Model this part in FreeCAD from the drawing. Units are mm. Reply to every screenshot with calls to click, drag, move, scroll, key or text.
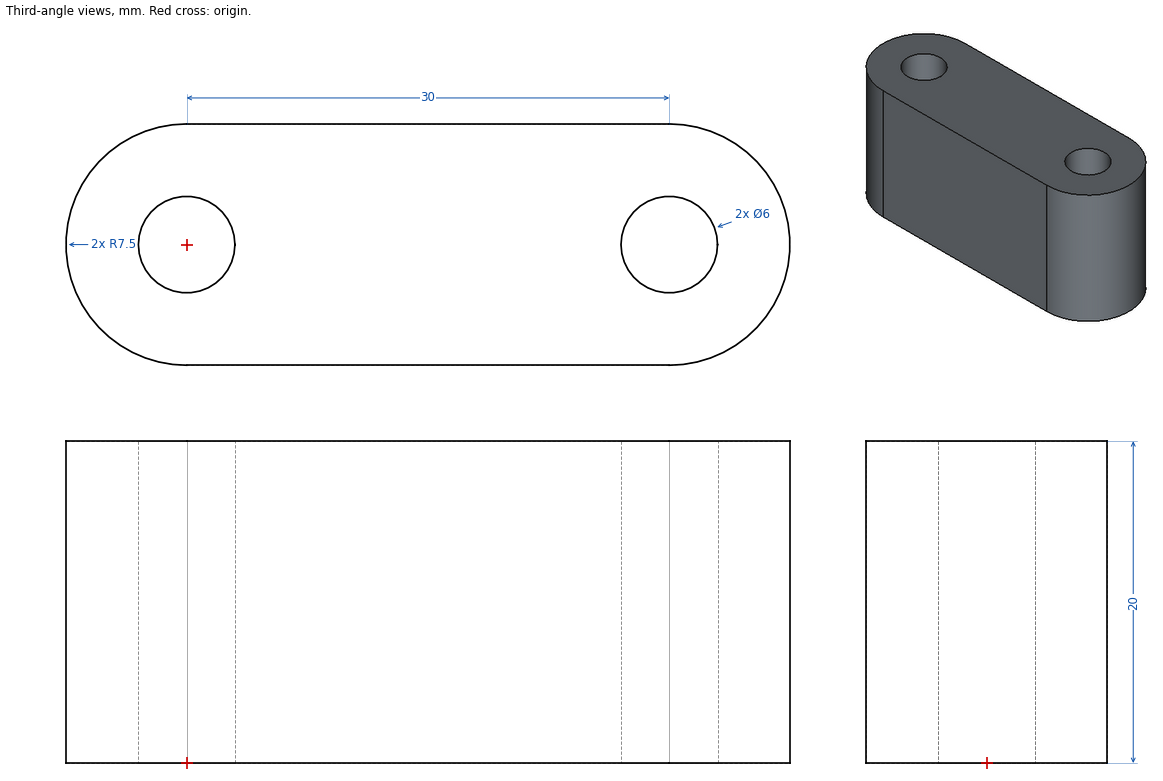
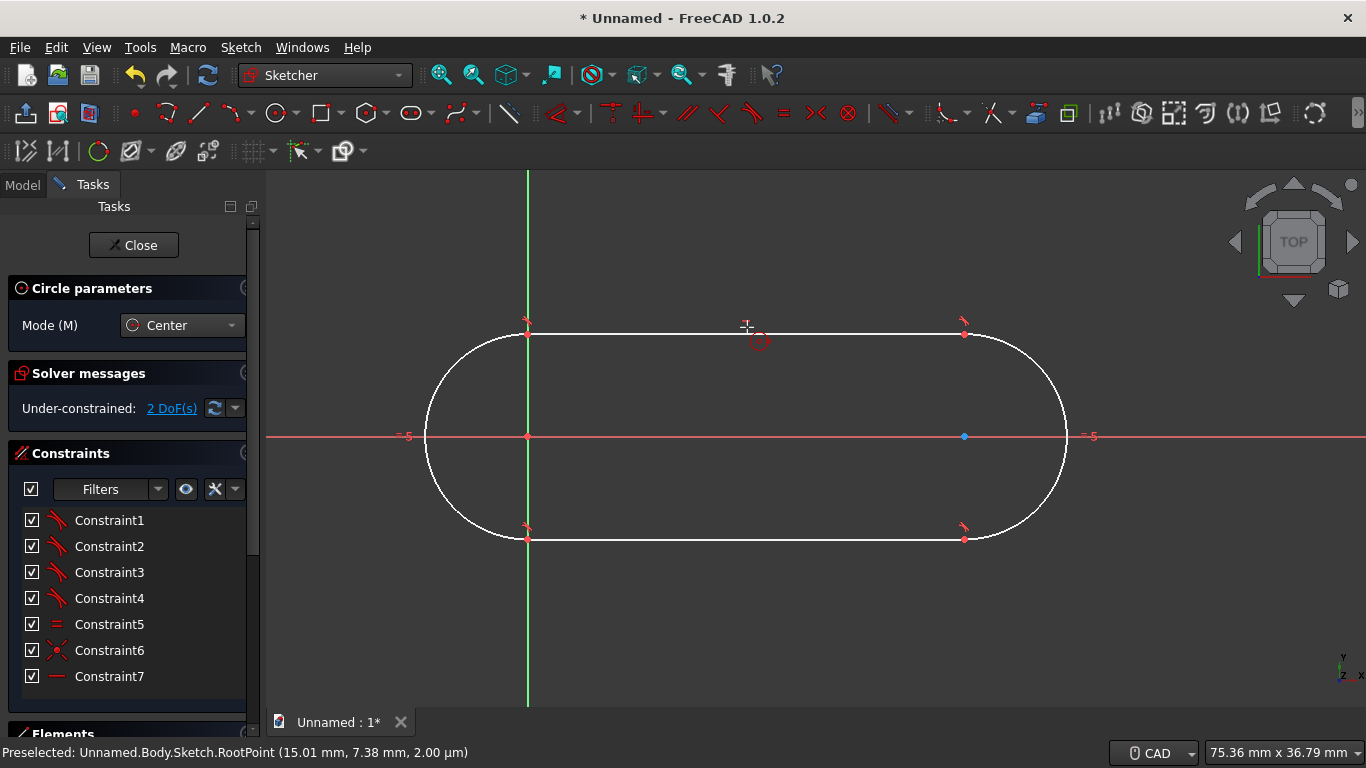
click(964, 437)
click(997, 406)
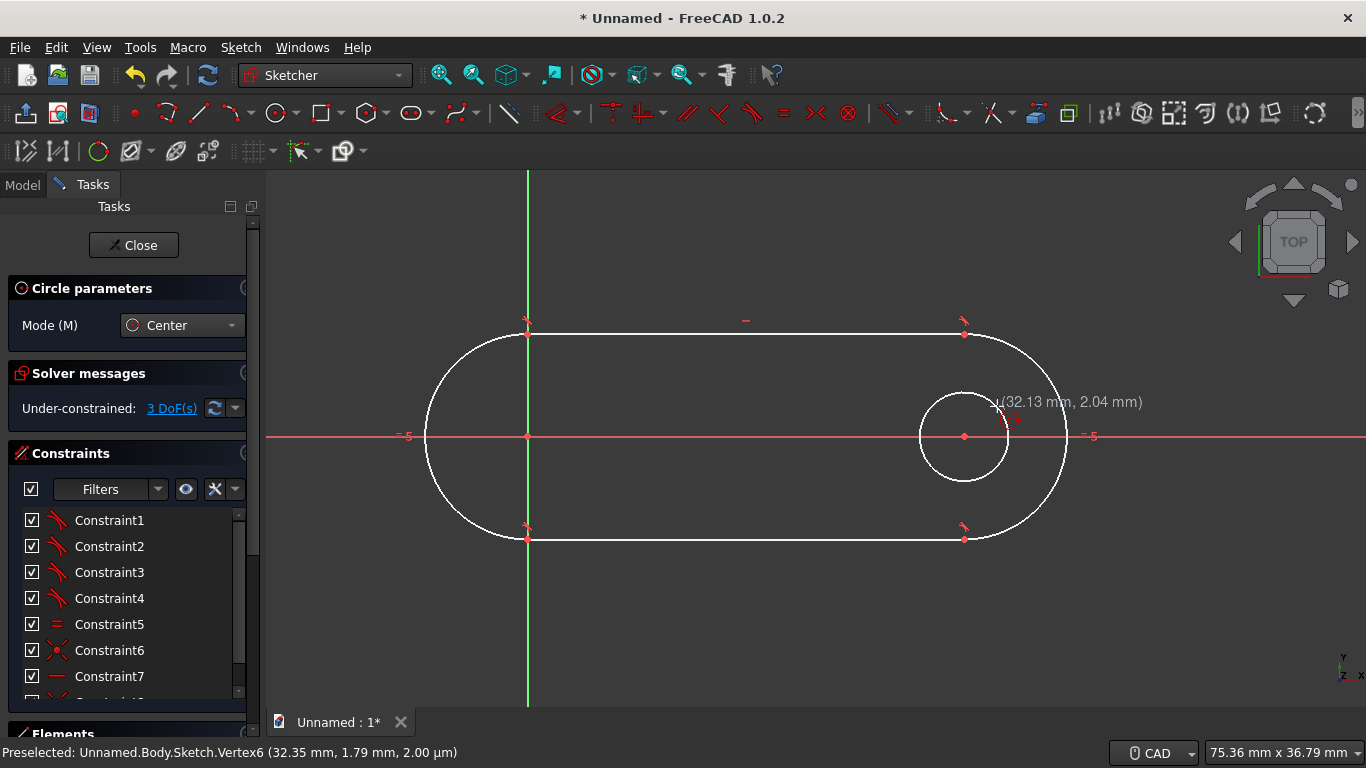
click(528, 437)
click(559, 406)
key(Escape)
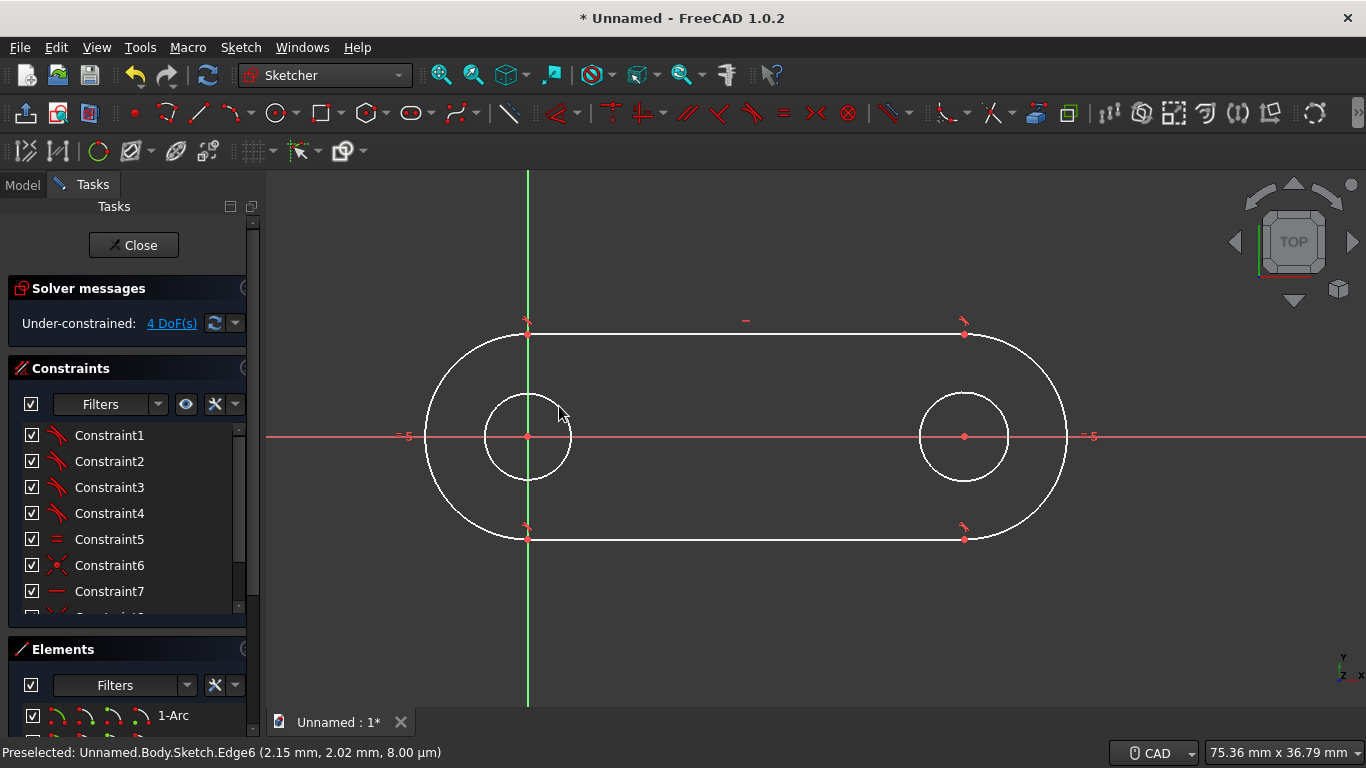
click(995, 405)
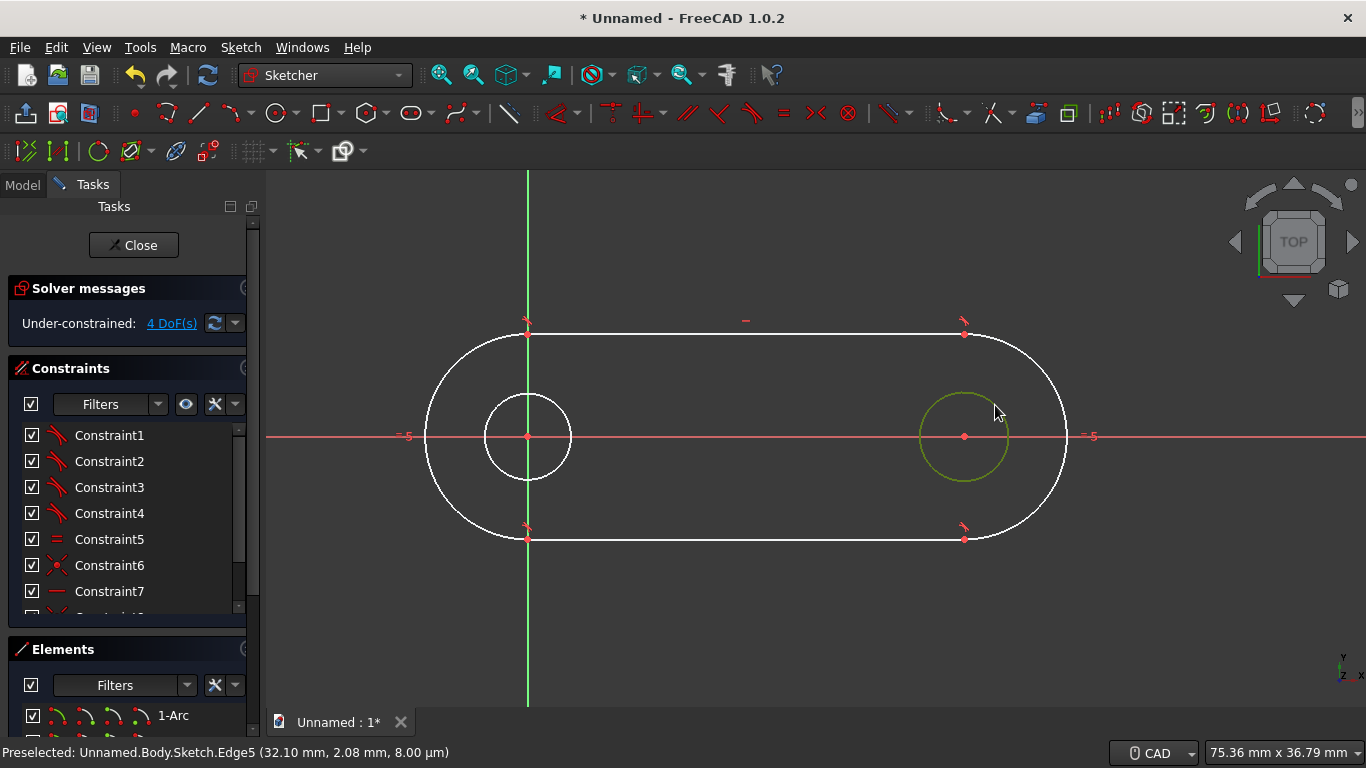
click(558, 406)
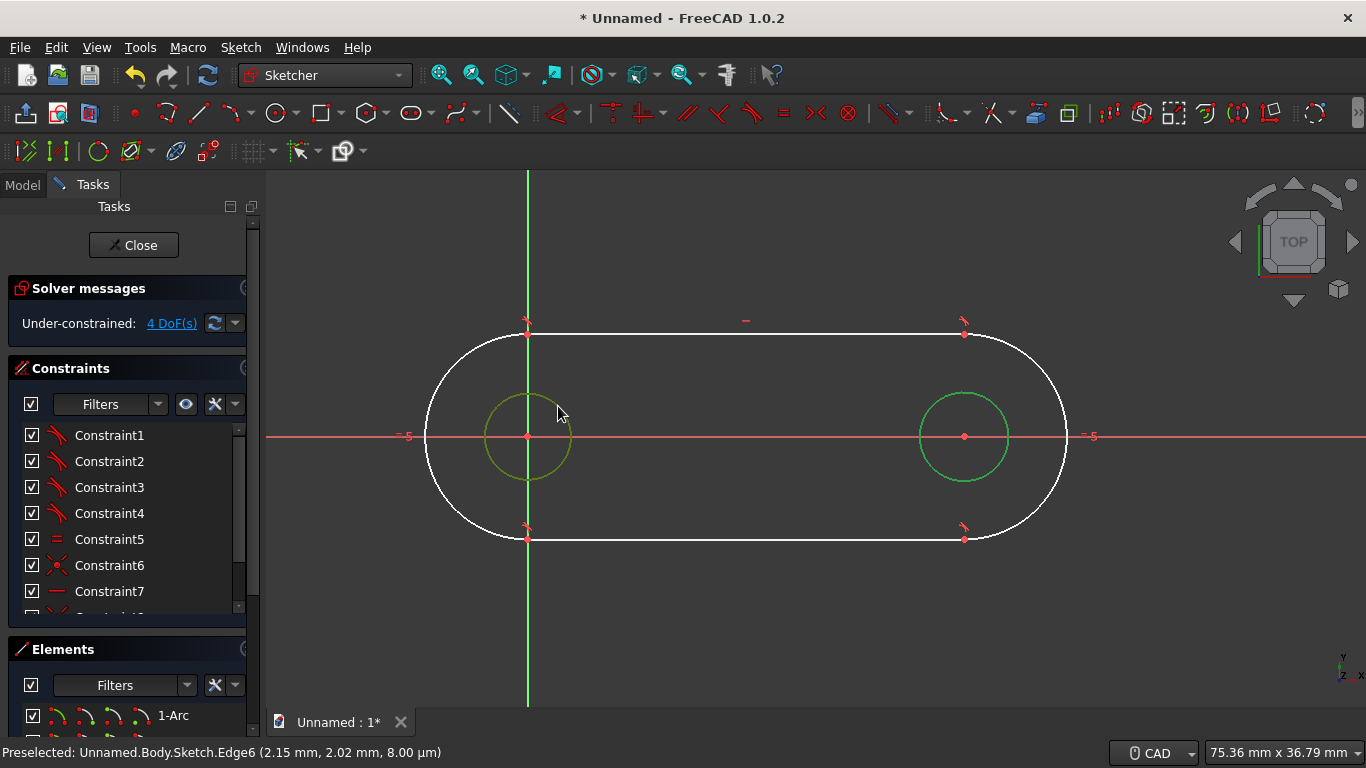
key(e)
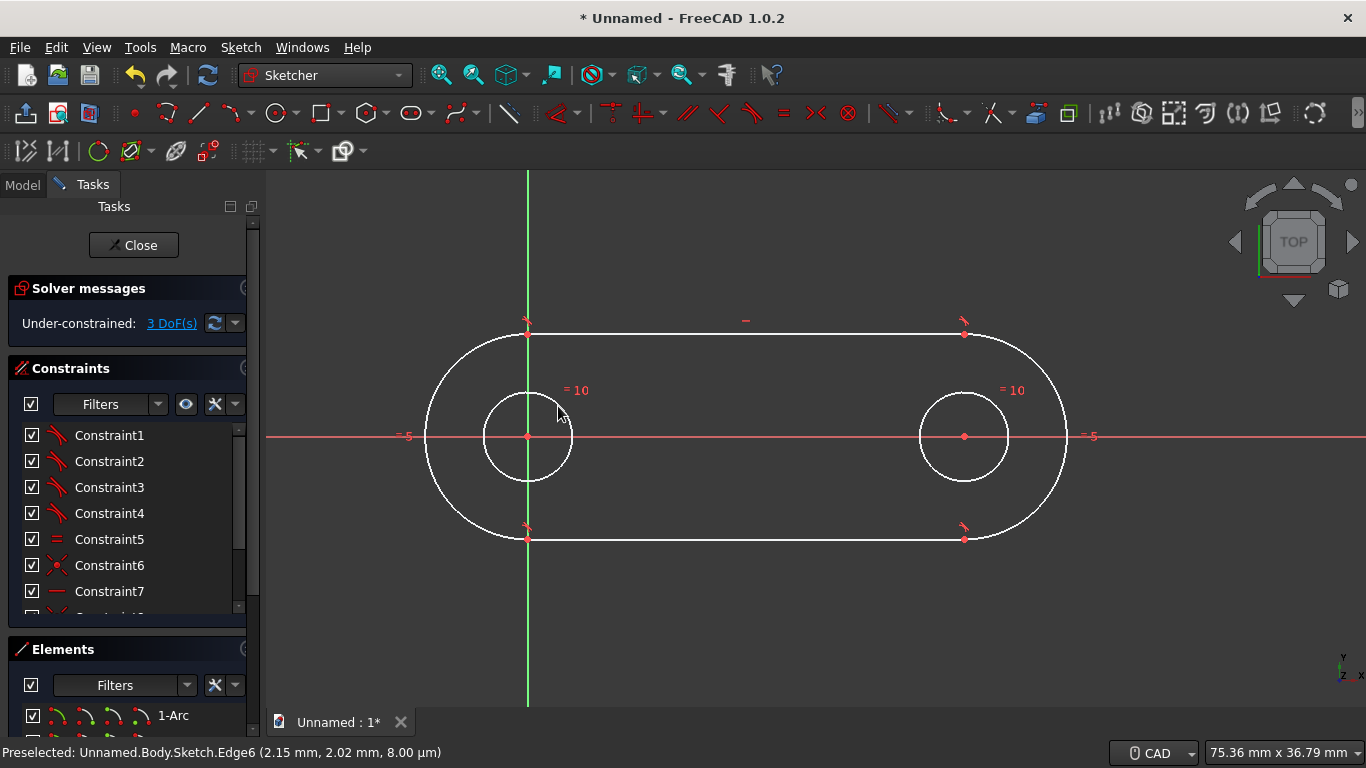
key(d)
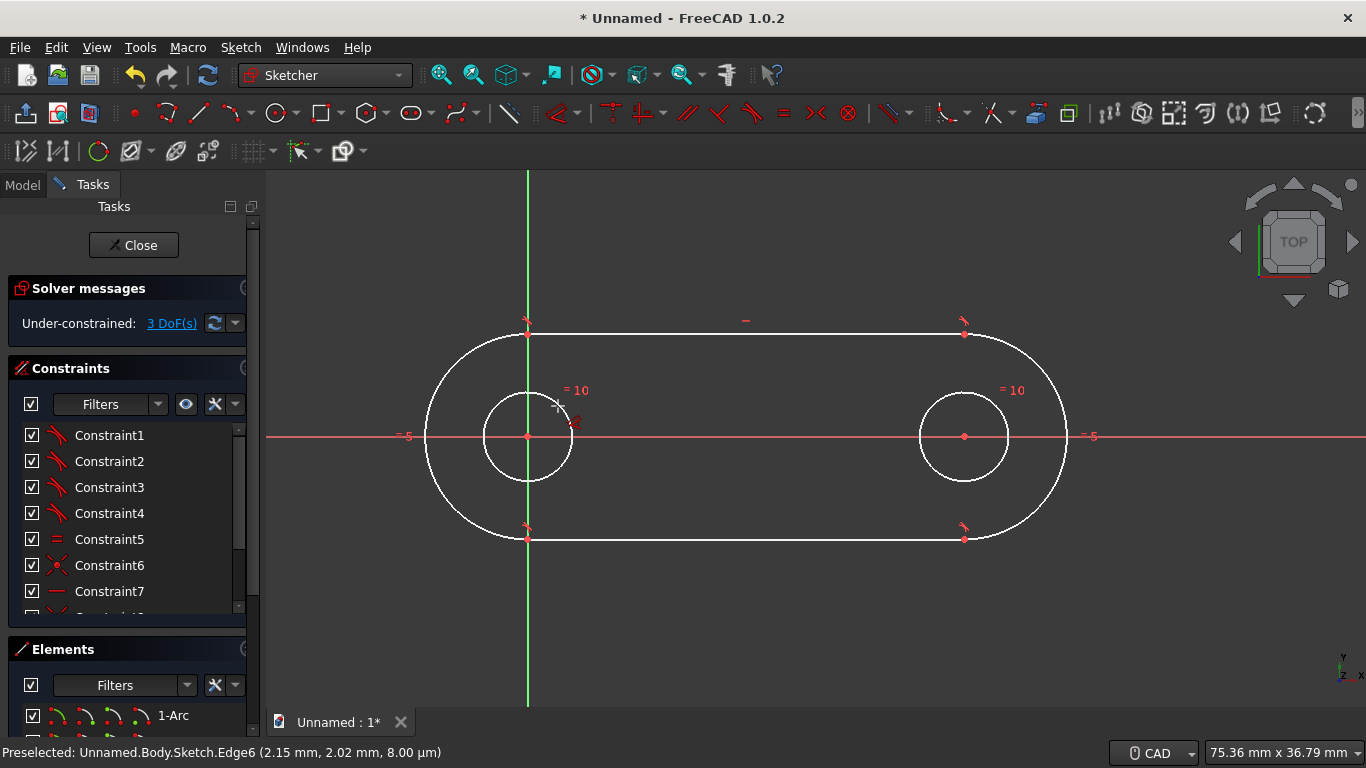
click(445, 376)
click(419, 357)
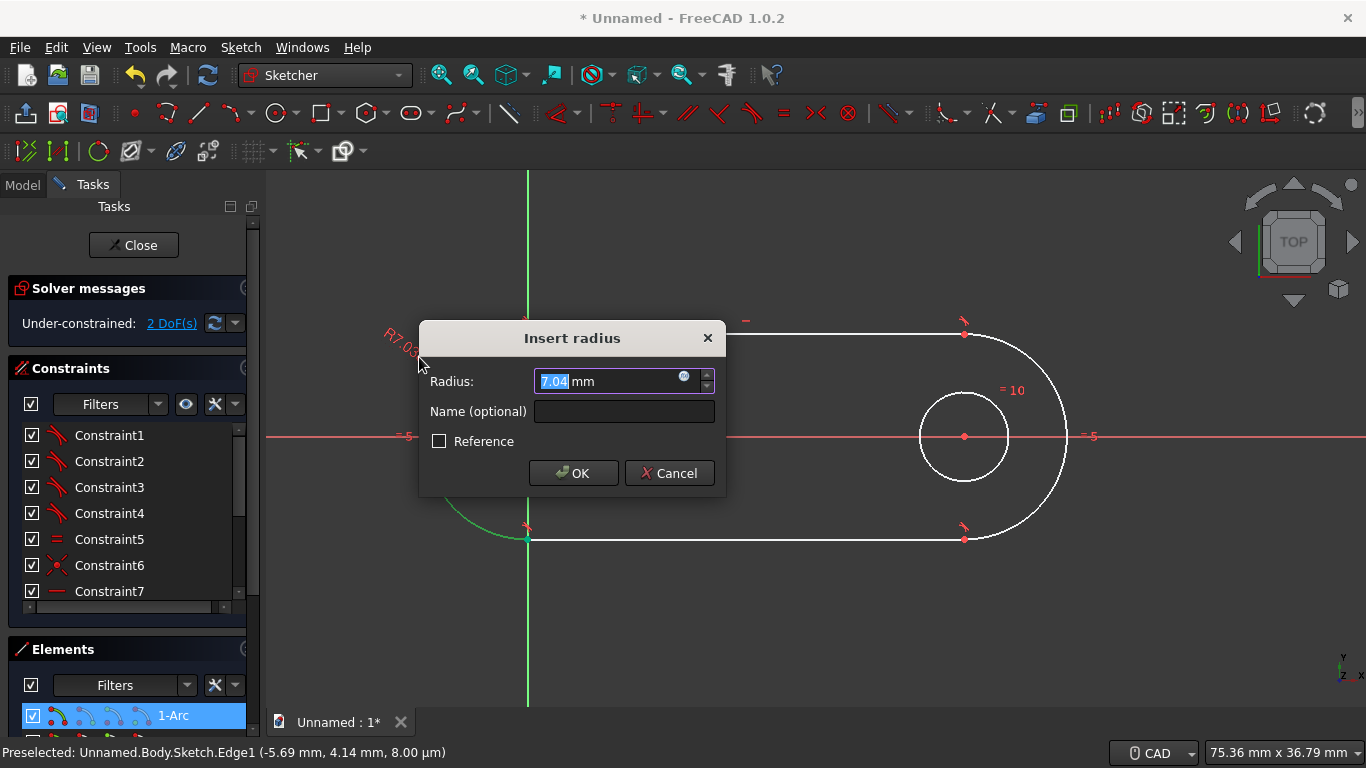
text(7.5)
key(Return)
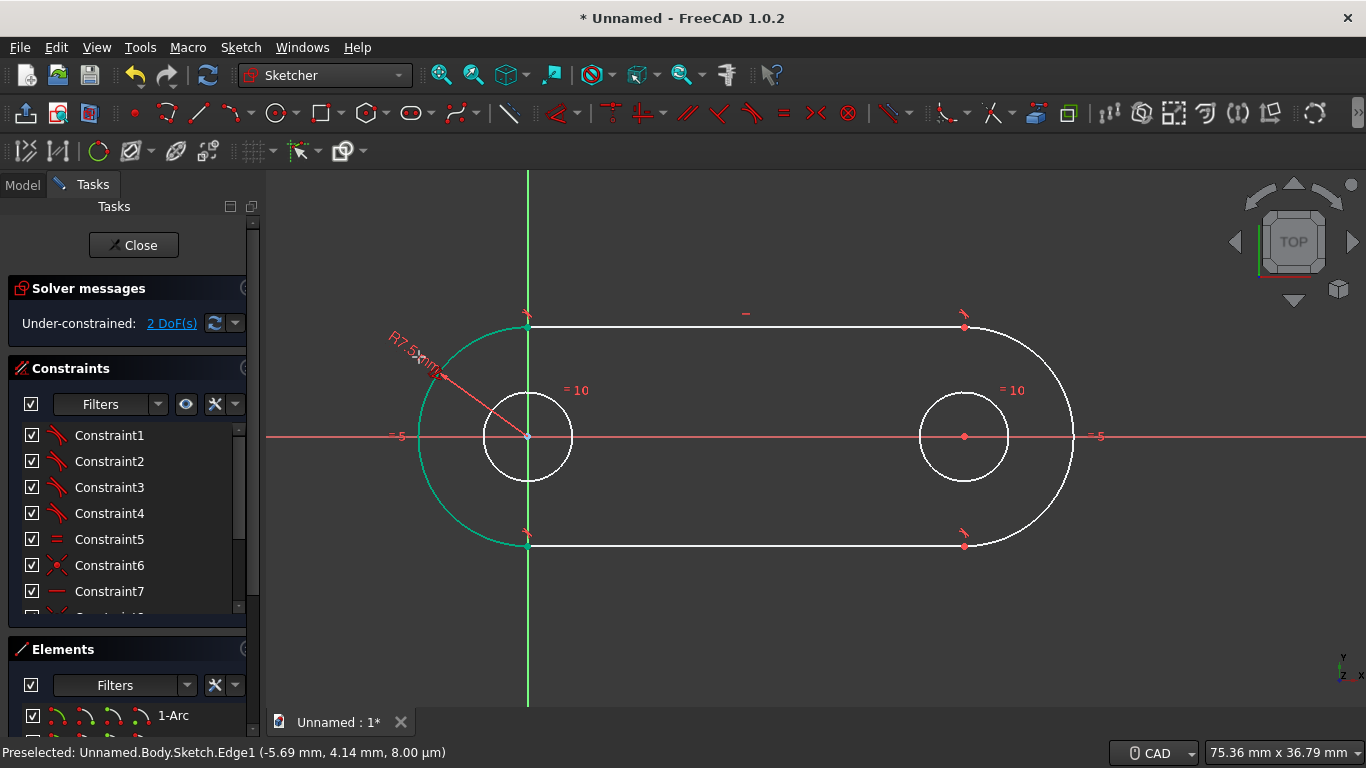
click(995, 405)
click(1017, 382)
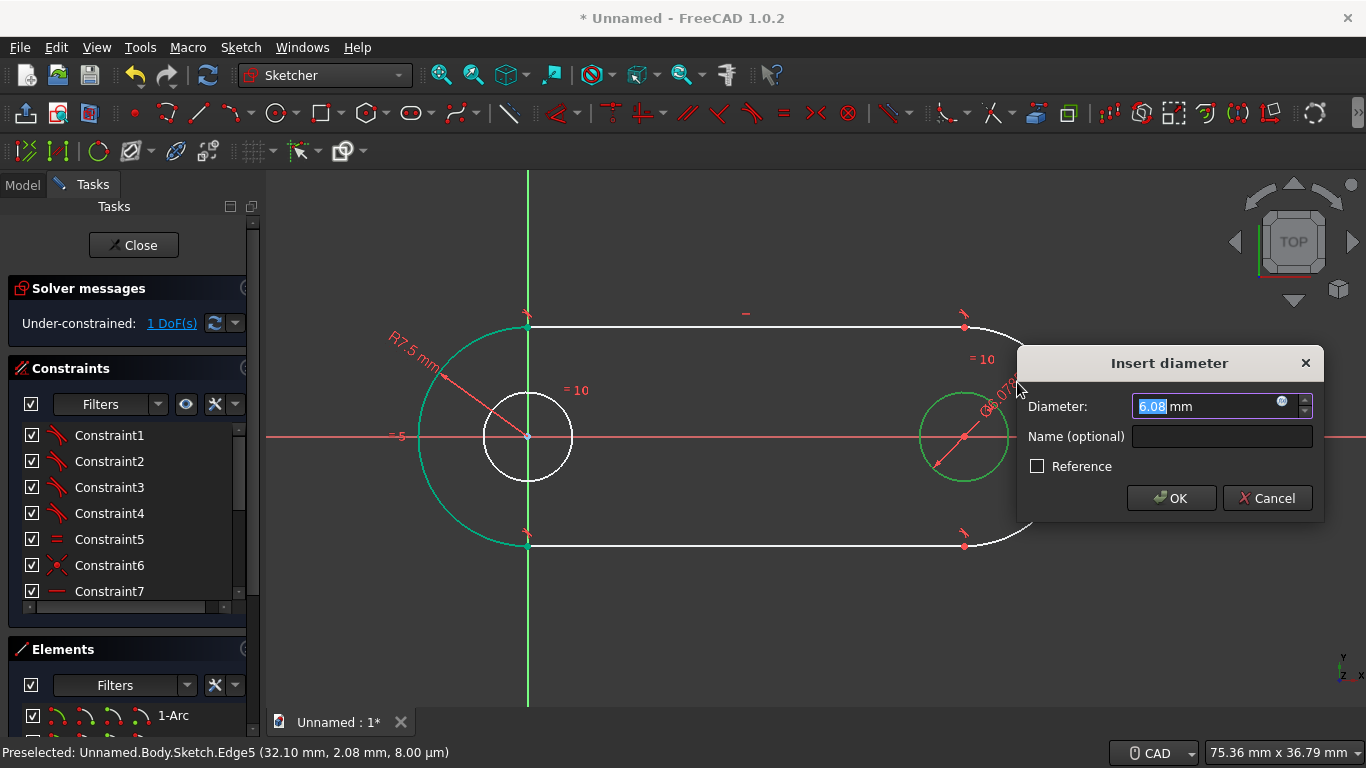
text(6)
key(Return)